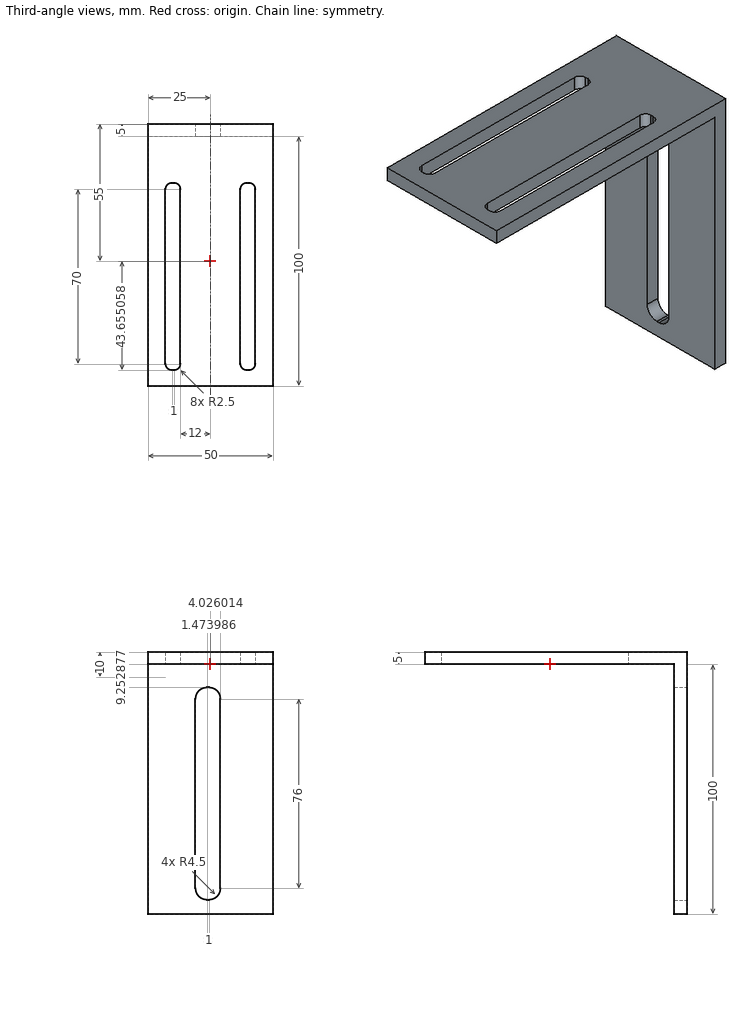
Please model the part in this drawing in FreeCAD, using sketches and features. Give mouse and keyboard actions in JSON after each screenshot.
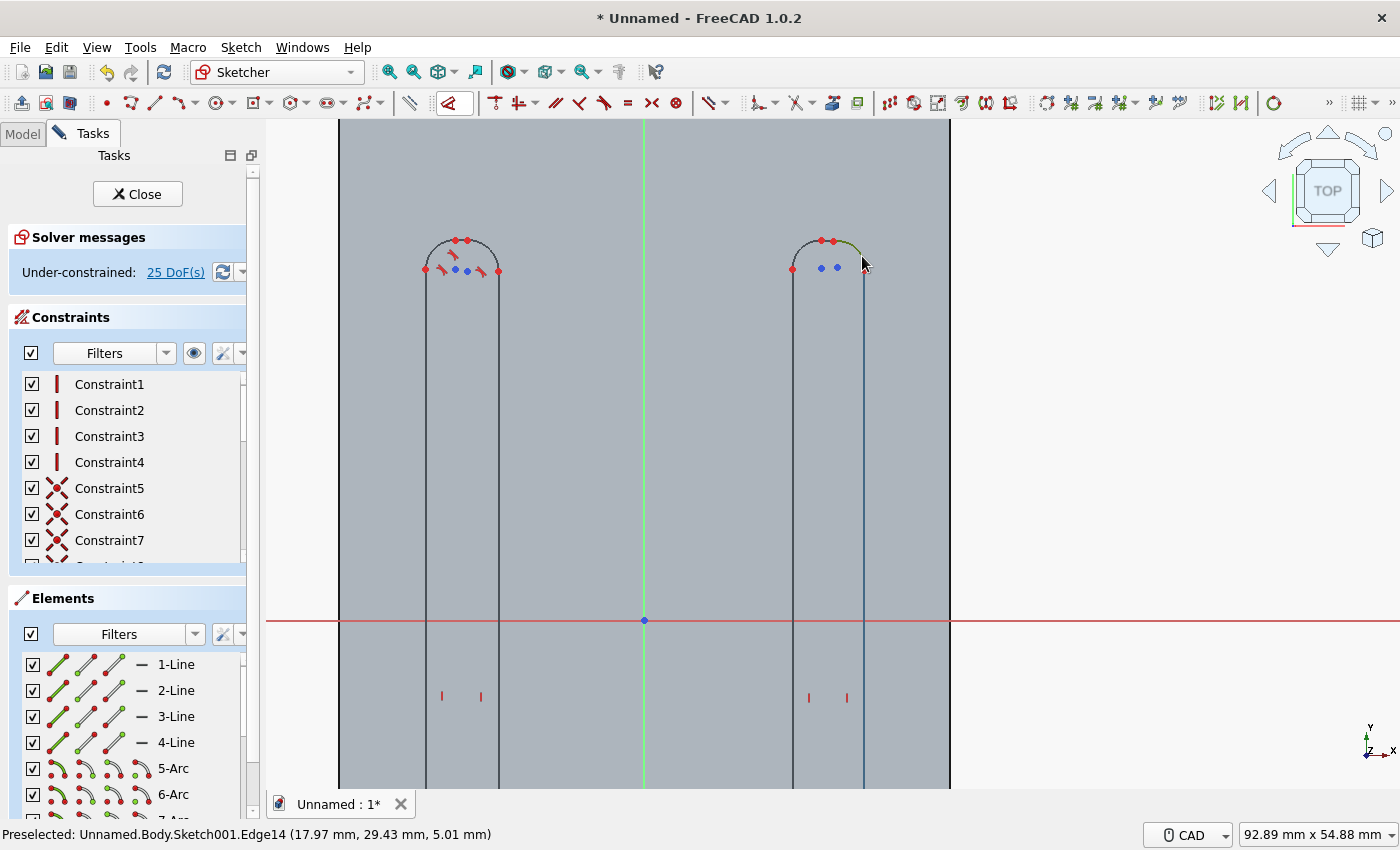
{"action": "left_click", "coordinate": [604, 104]}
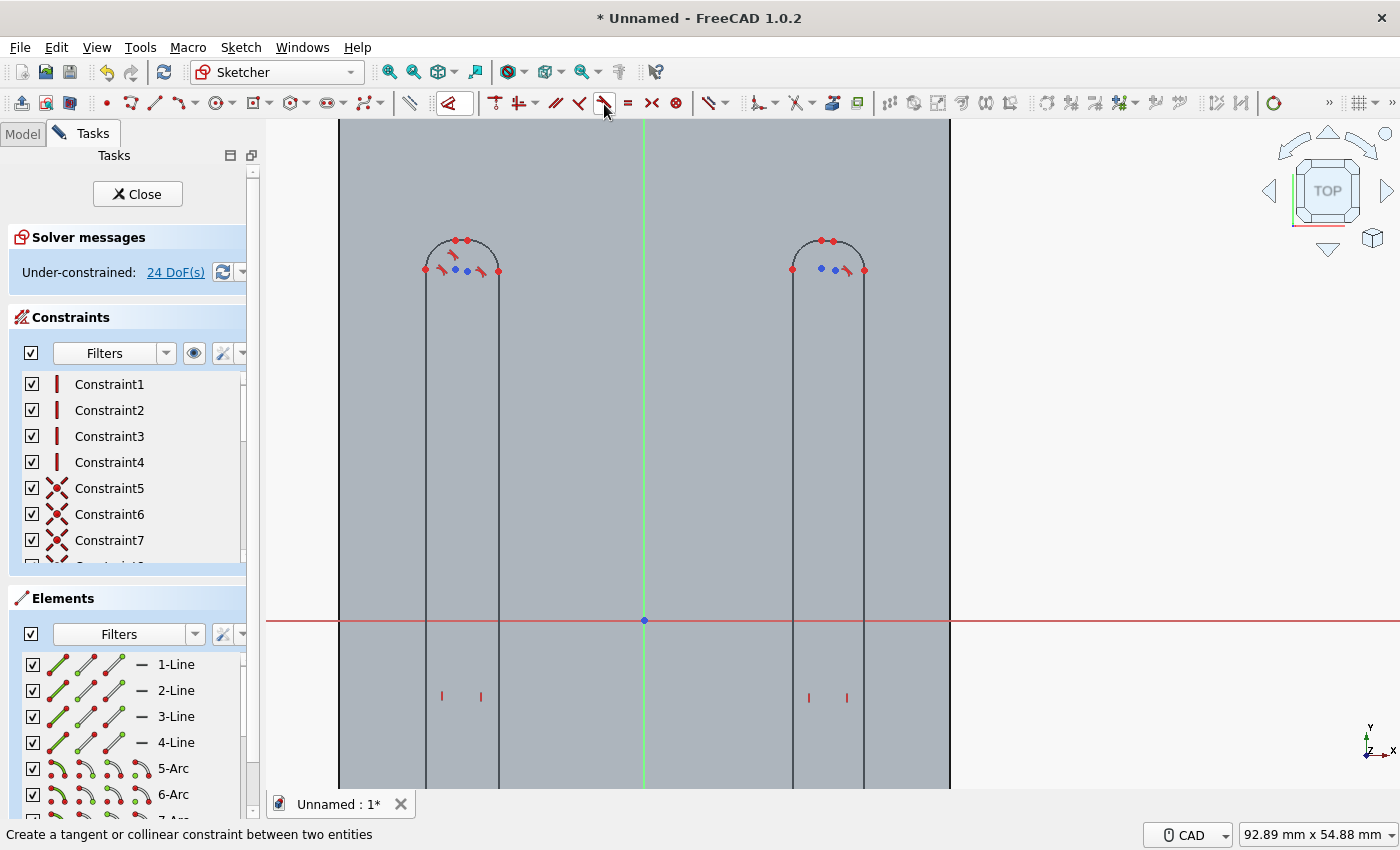
{"action": "scroll", "coordinate": [827, 241], "scroll_direction": "up", "scroll_amount": 5}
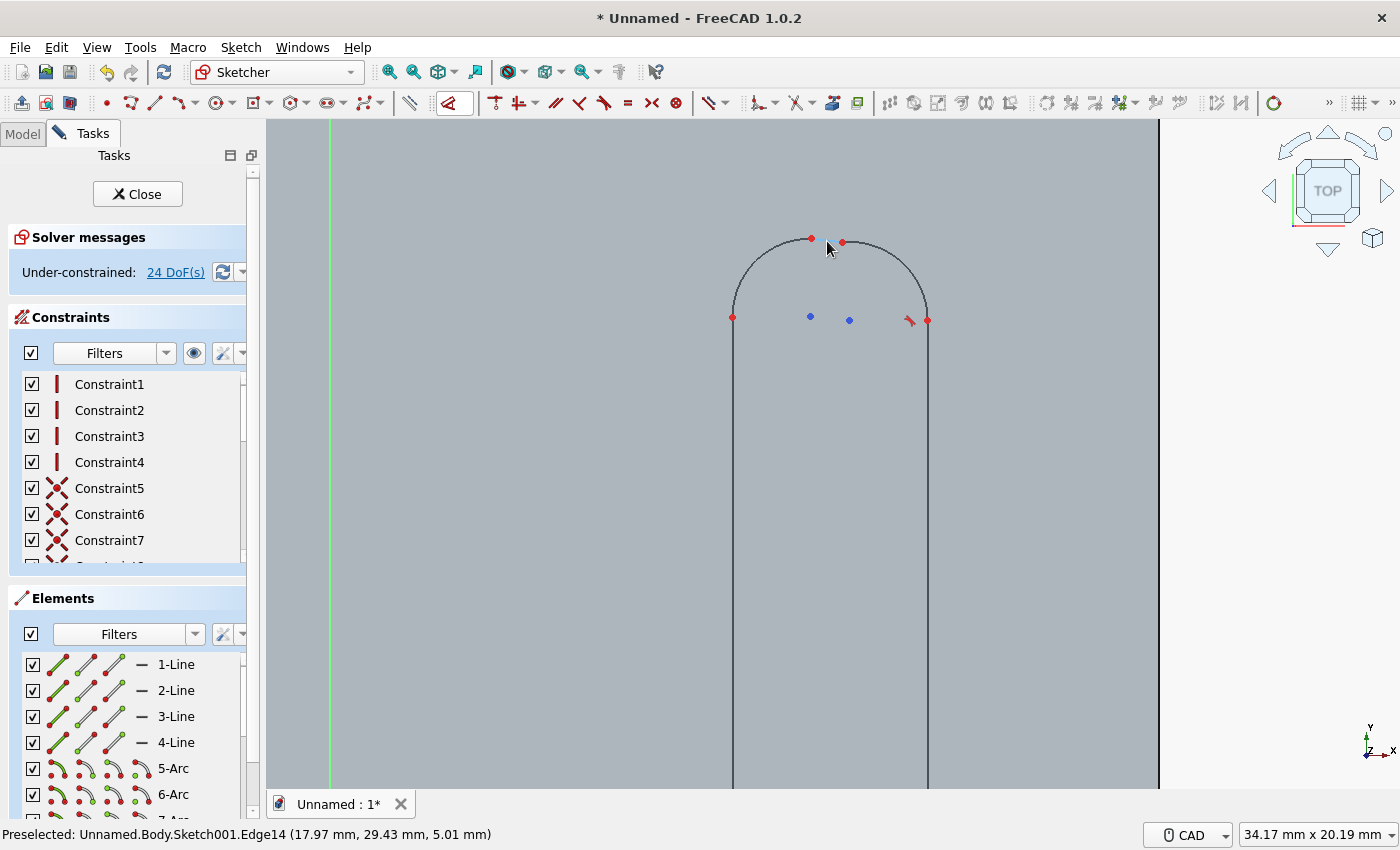
{"action": "left_click", "coordinate": [827, 240]}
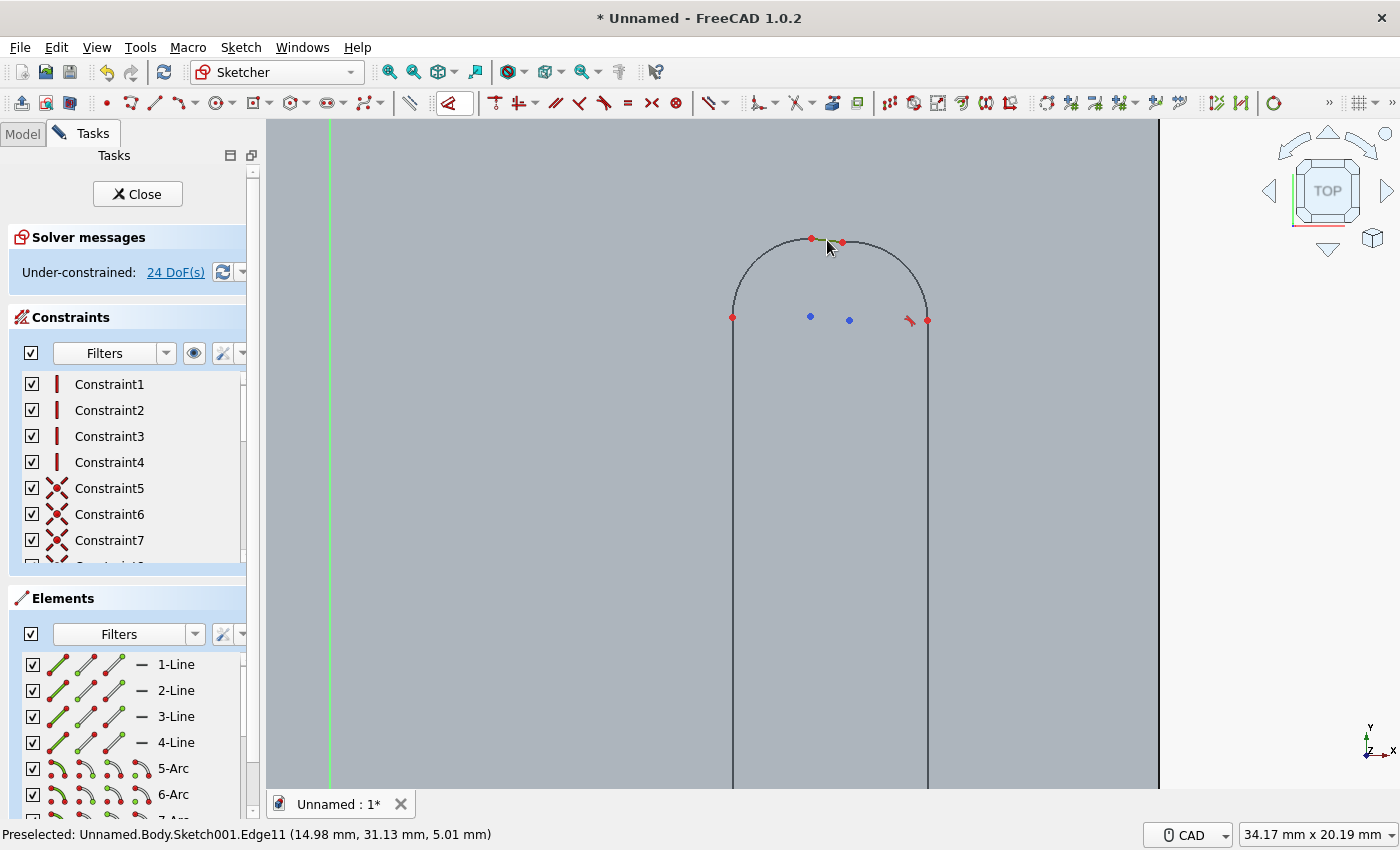
{"action": "left_click", "coordinate": [918, 283]}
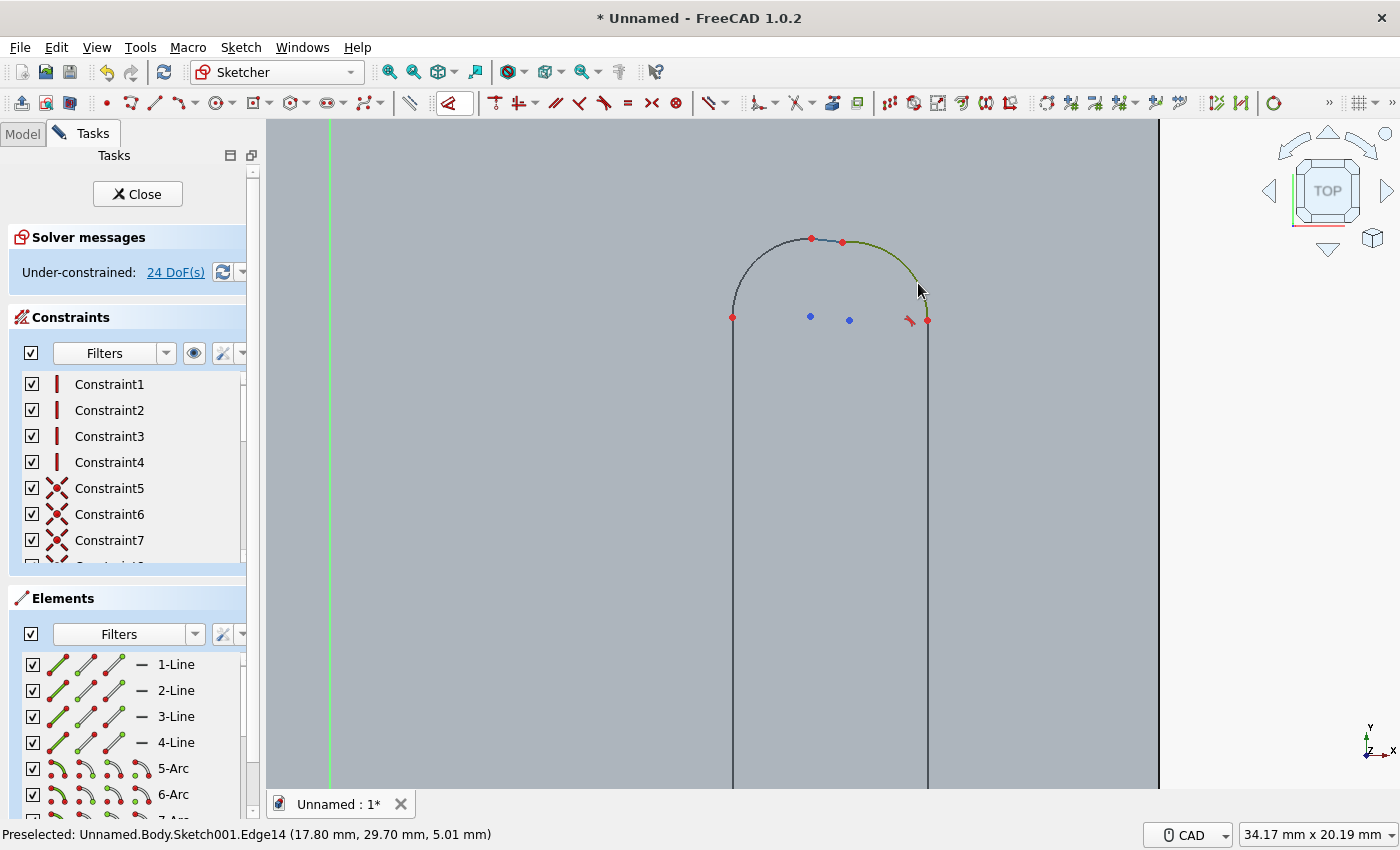
{"action": "left_click", "coordinate": [604, 104]}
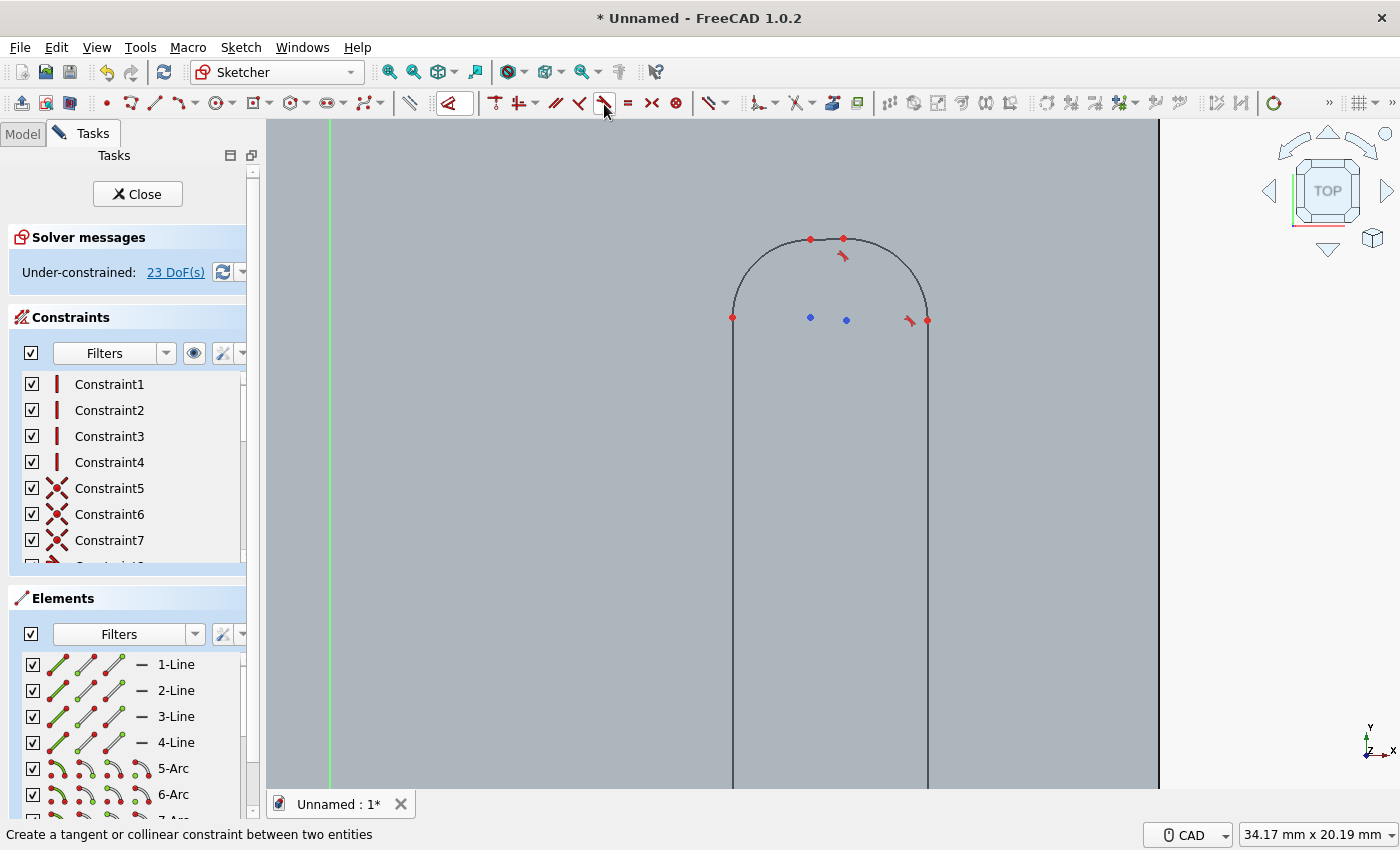
{"action": "scroll", "coordinate": [834, 239], "scroll_direction": "up", "scroll_amount": 2}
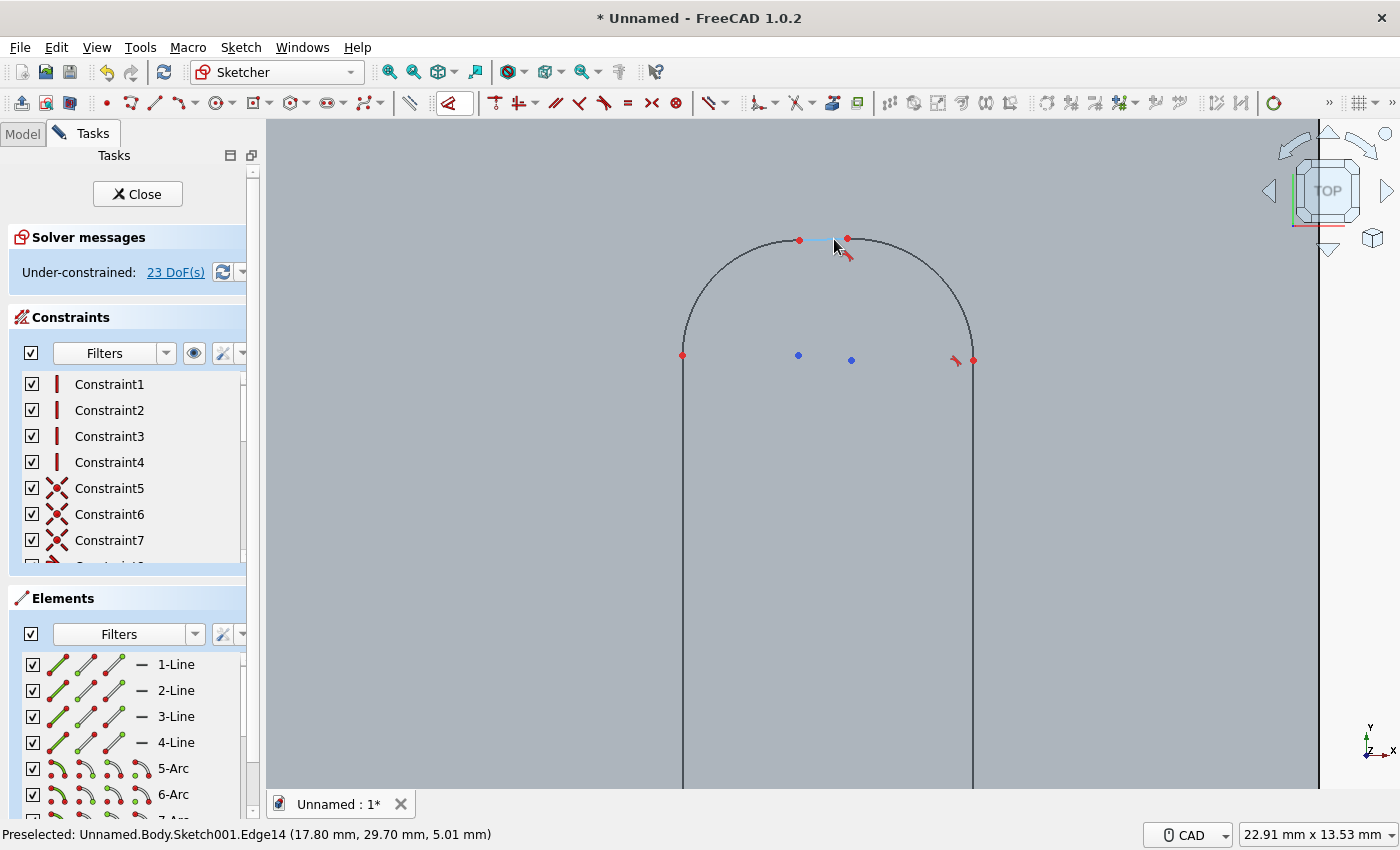
{"action": "left_click", "coordinate": [833, 239]}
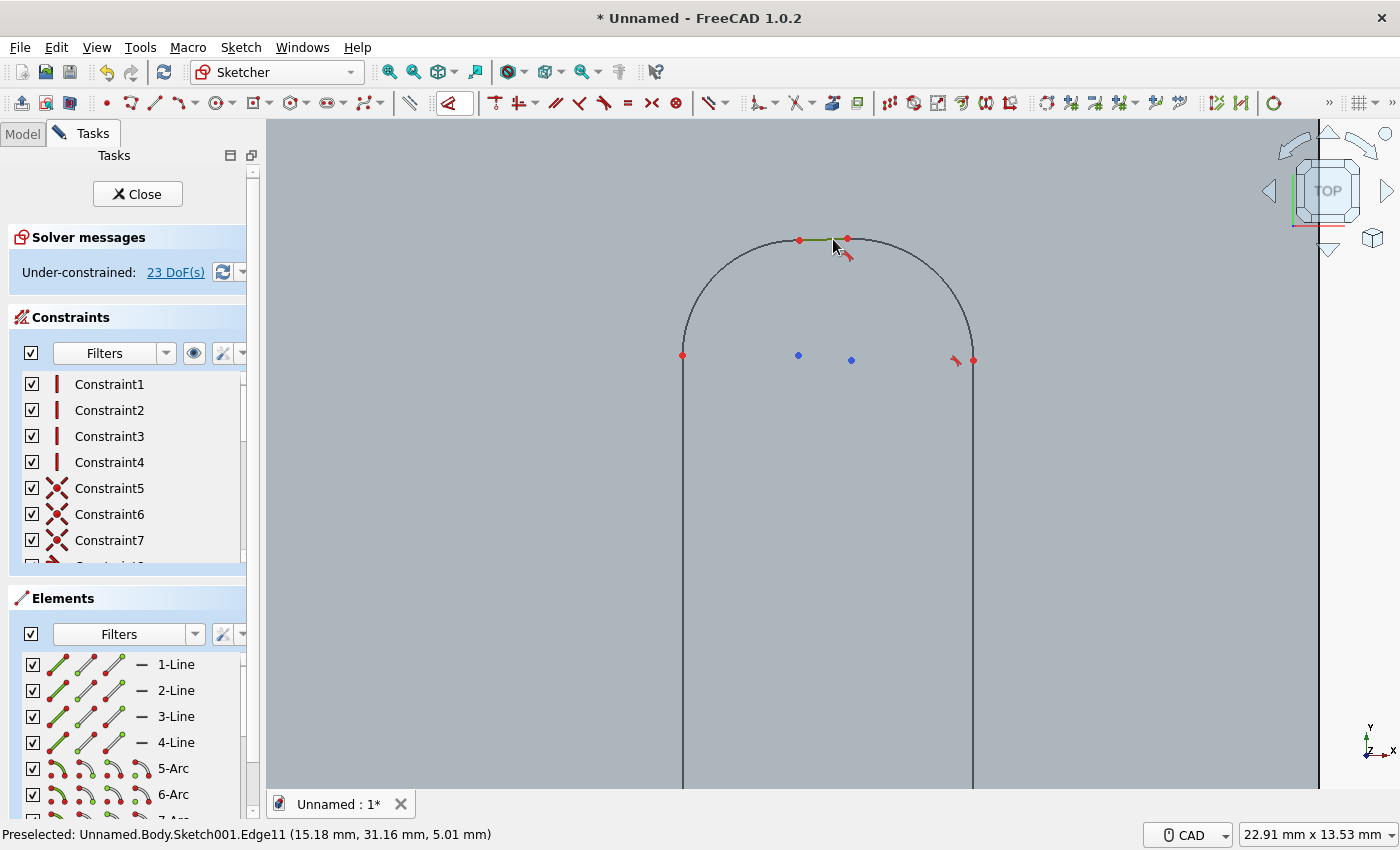
{"action": "scroll", "coordinate": [850, 251], "scroll_direction": "down", "scroll_amount": 11}